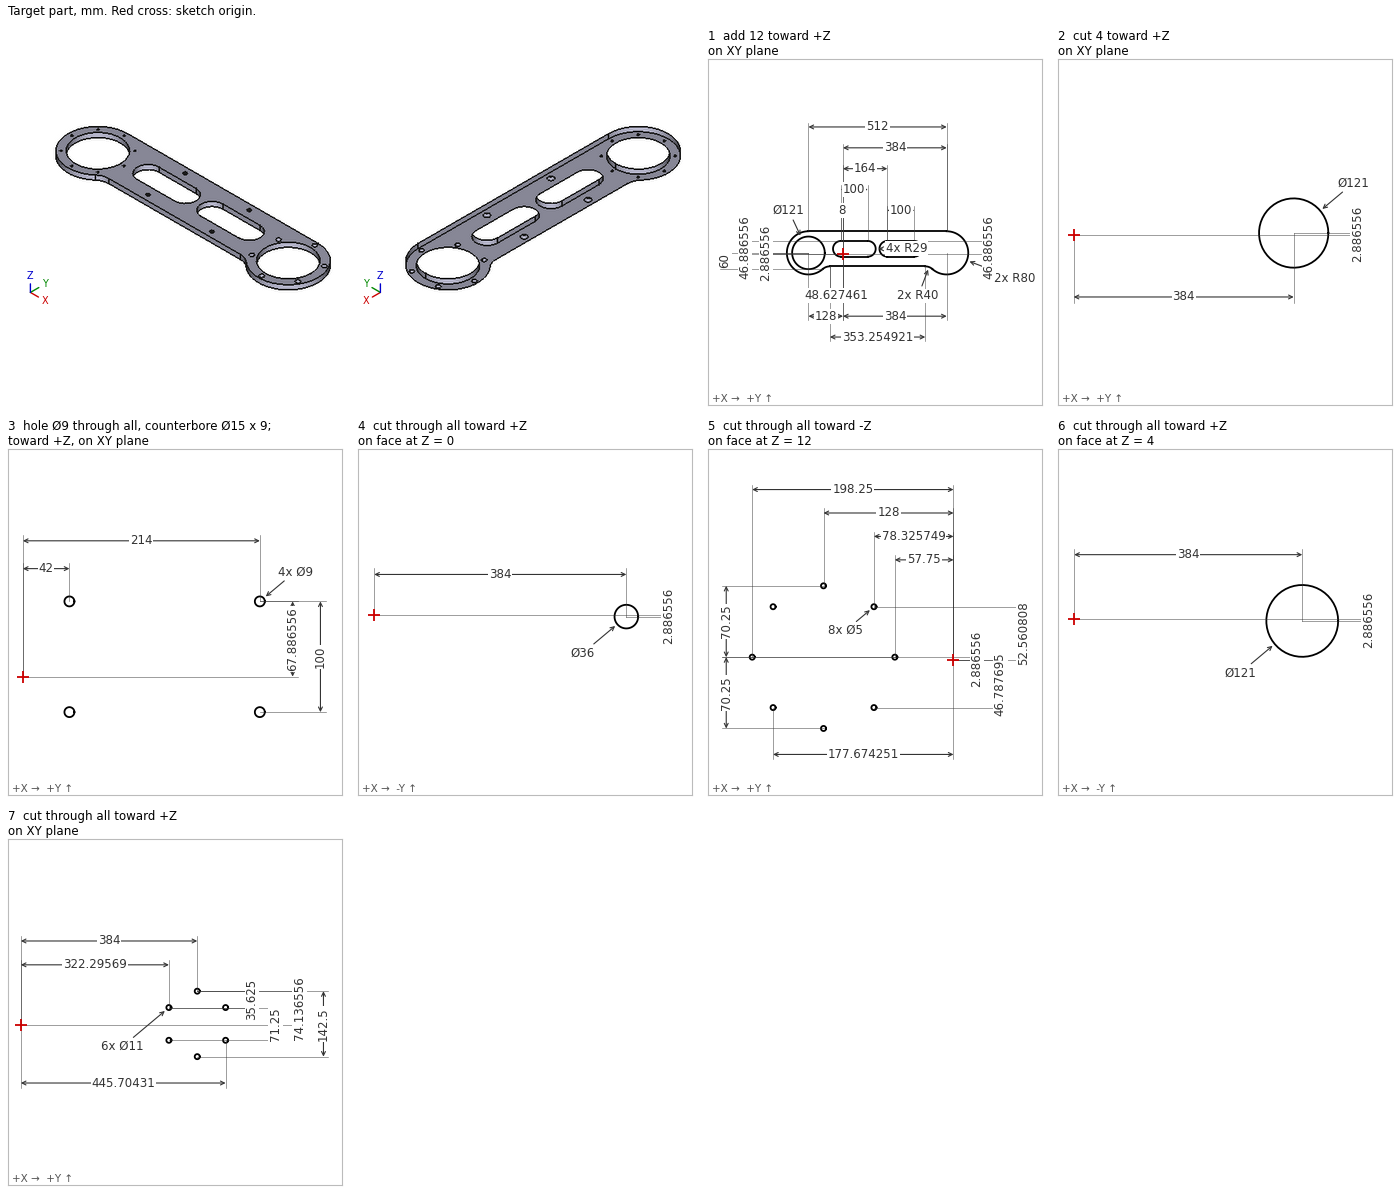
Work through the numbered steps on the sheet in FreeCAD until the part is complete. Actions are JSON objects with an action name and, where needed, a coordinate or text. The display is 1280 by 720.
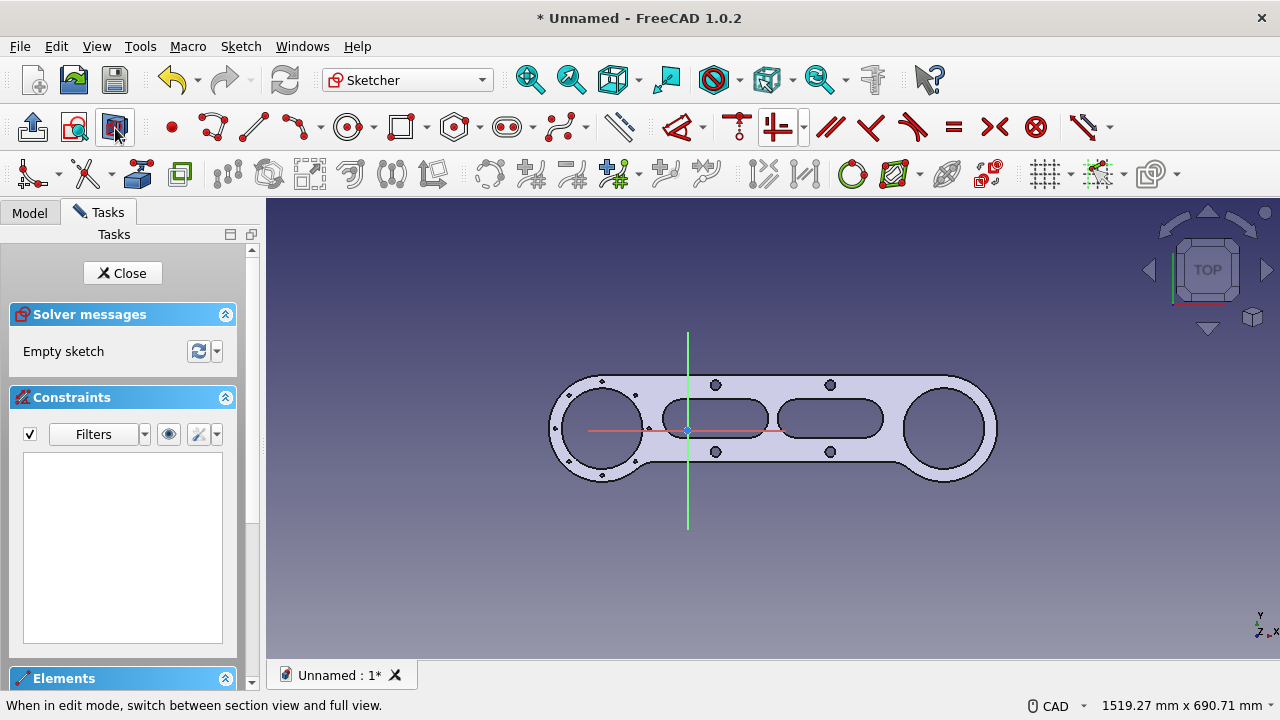
{"action": "scroll", "coordinate": [1083, 429], "scroll_direction": "up", "scroll_amount": 5}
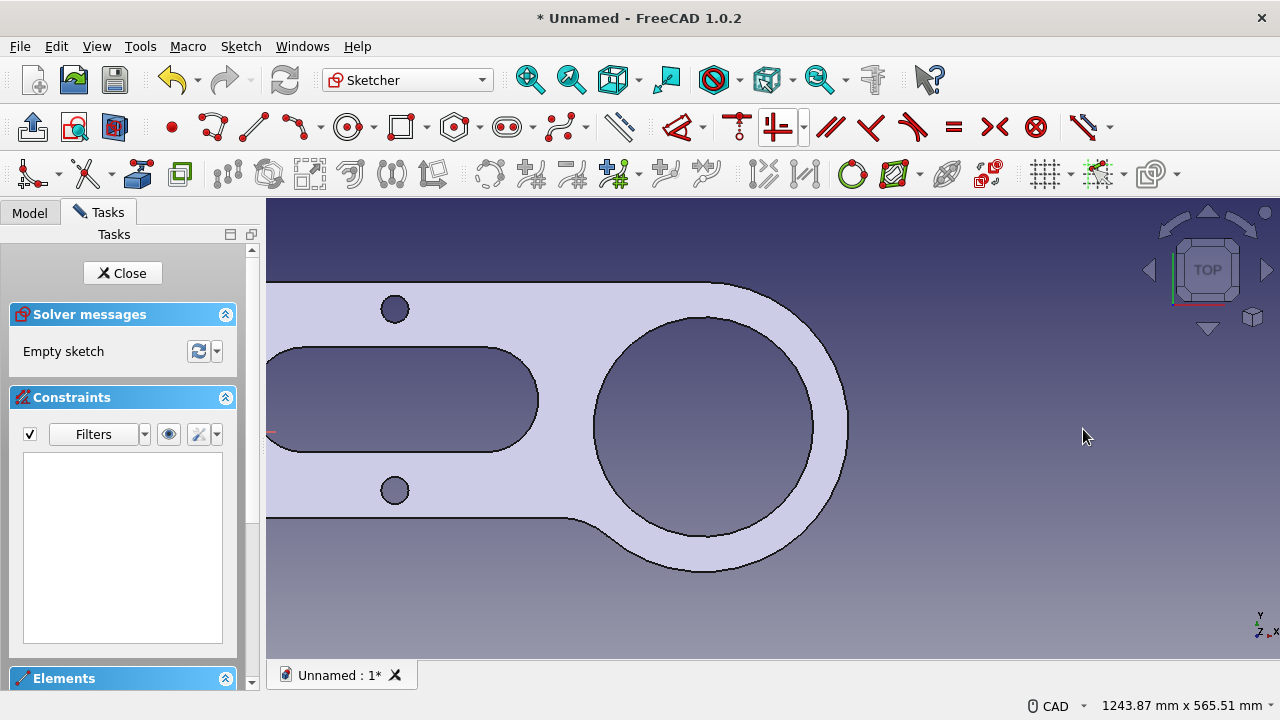
{"action": "left_click", "coordinate": [348, 128]}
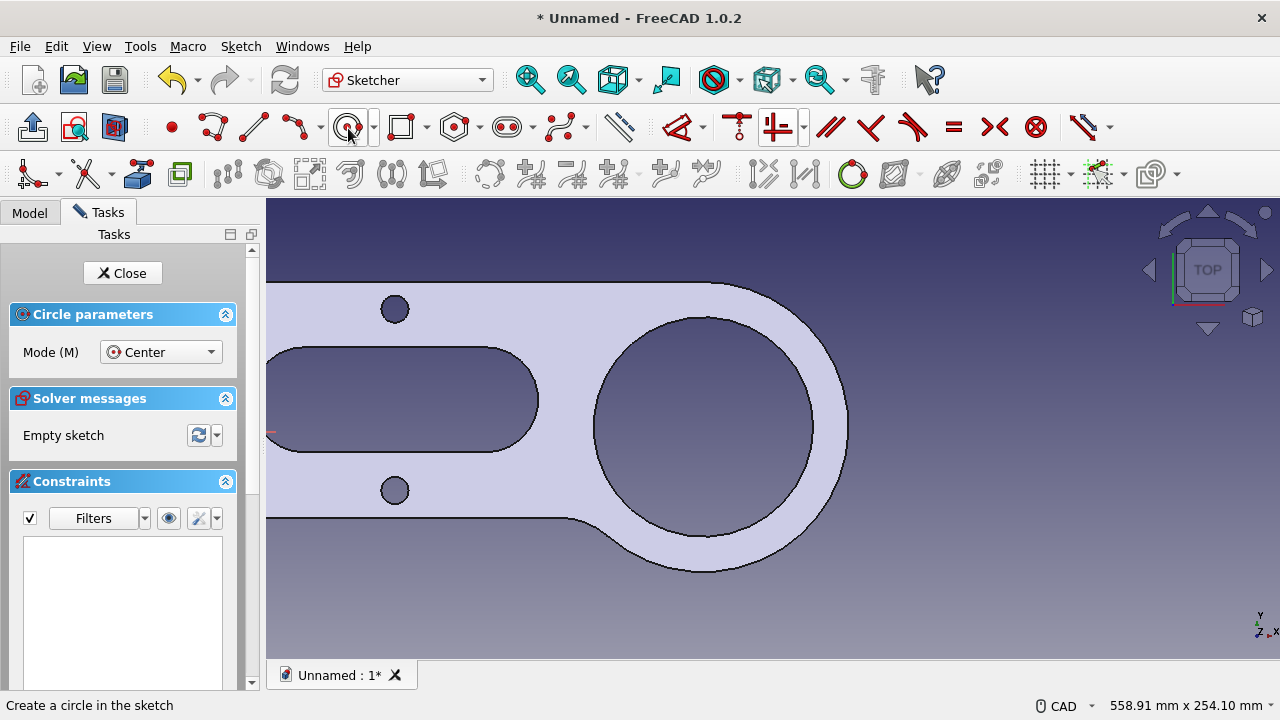
{"action": "scroll", "coordinate": [703, 298], "scroll_direction": "up", "scroll_amount": 5}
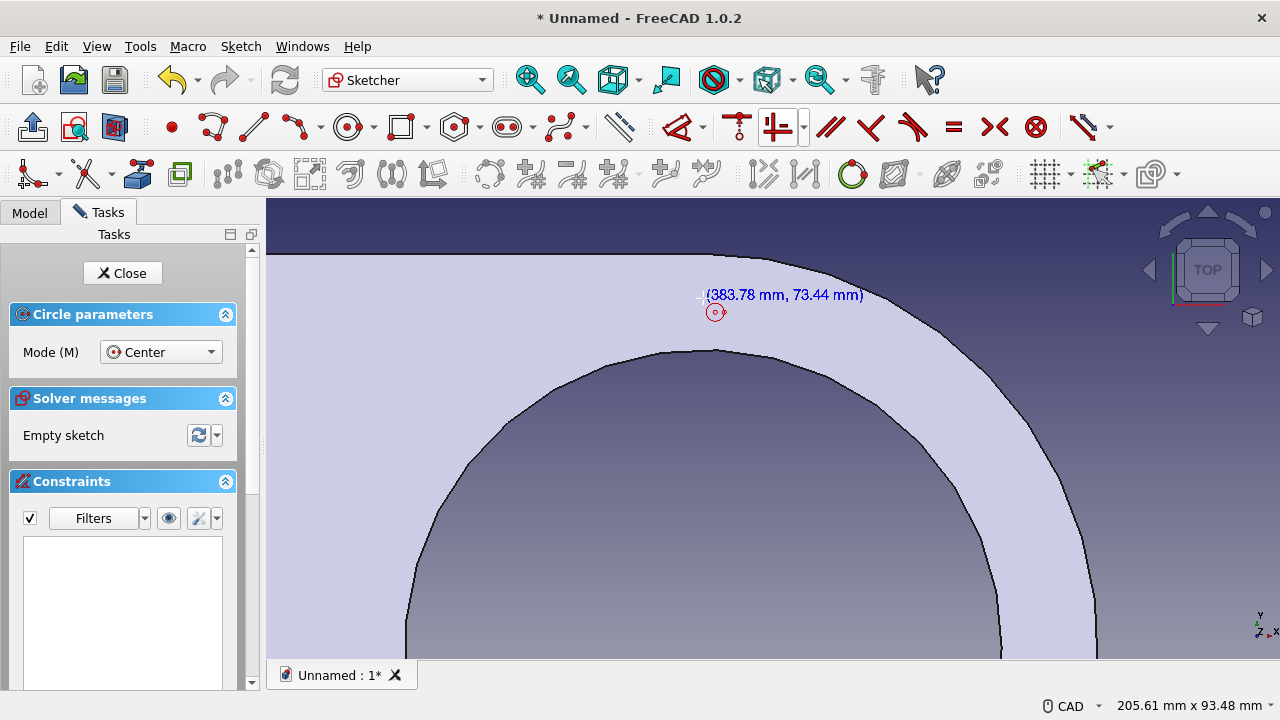
{"action": "left_click", "coordinate": [703, 297]}
{"action": "left_click", "coordinate": [723, 278]}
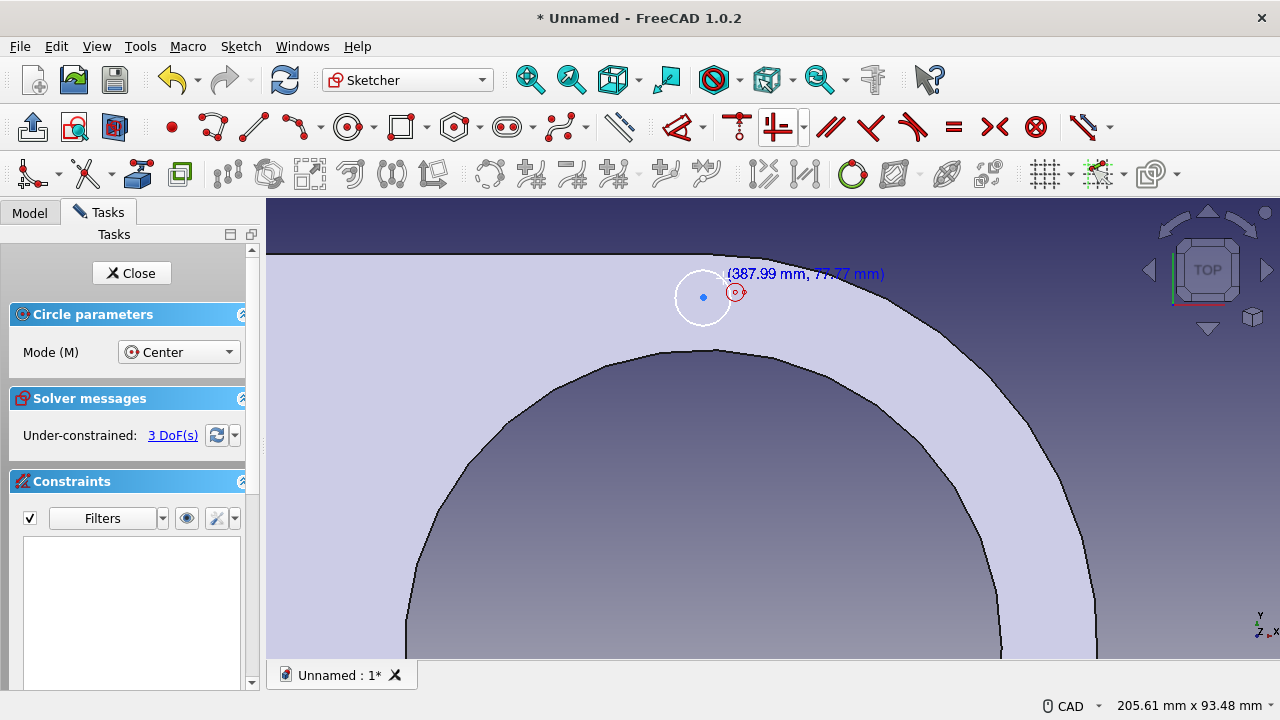
{"action": "left_click", "coordinate": [399, 473]}
{"action": "left_click", "coordinate": [418, 453]}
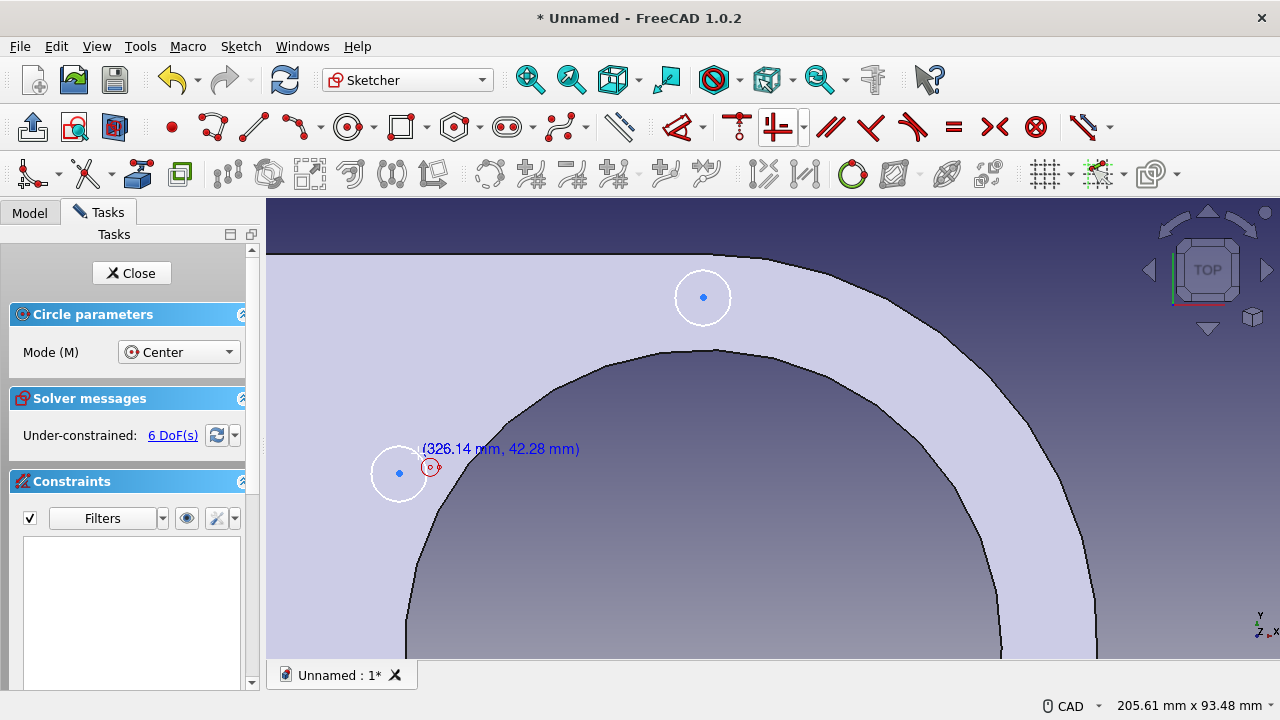
{"action": "scroll", "coordinate": [705, 301], "scroll_direction": "down", "scroll_amount": 5}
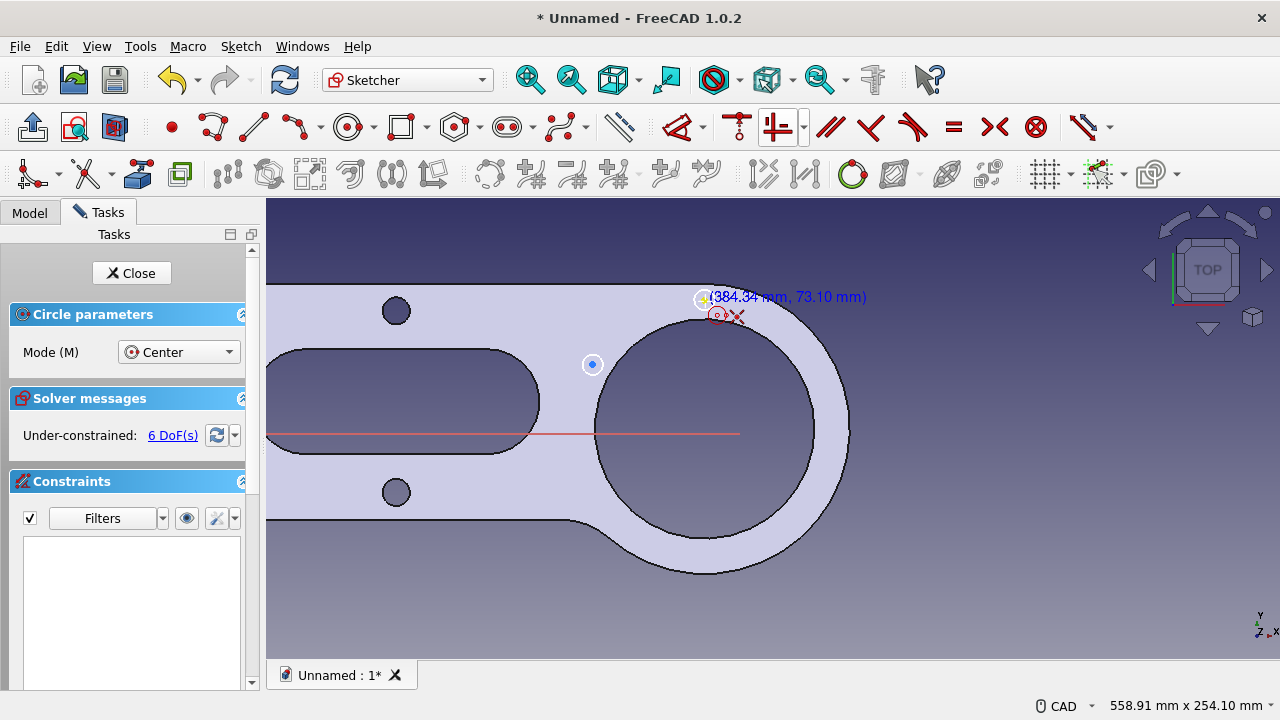
{"action": "scroll", "coordinate": [593, 494], "scroll_direction": "up", "scroll_amount": 5}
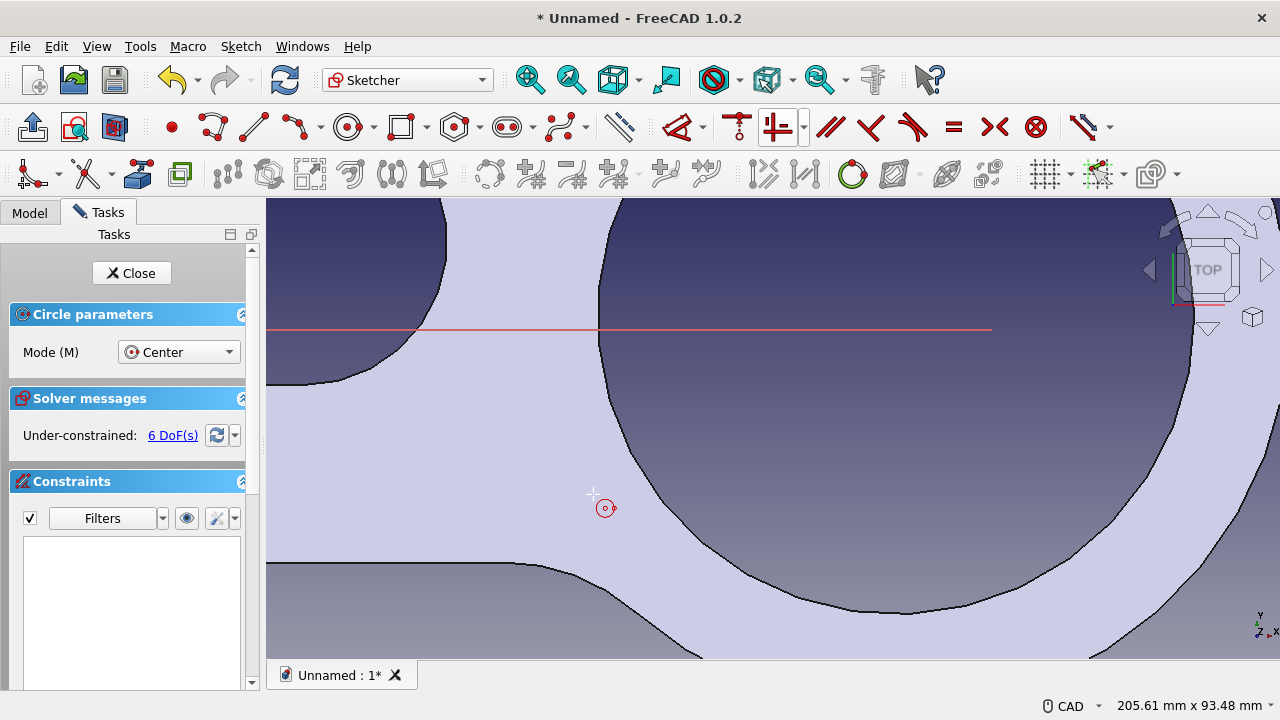
{"action": "left_click", "coordinate": [592, 492]}
{"action": "left_click", "coordinate": [611, 472]}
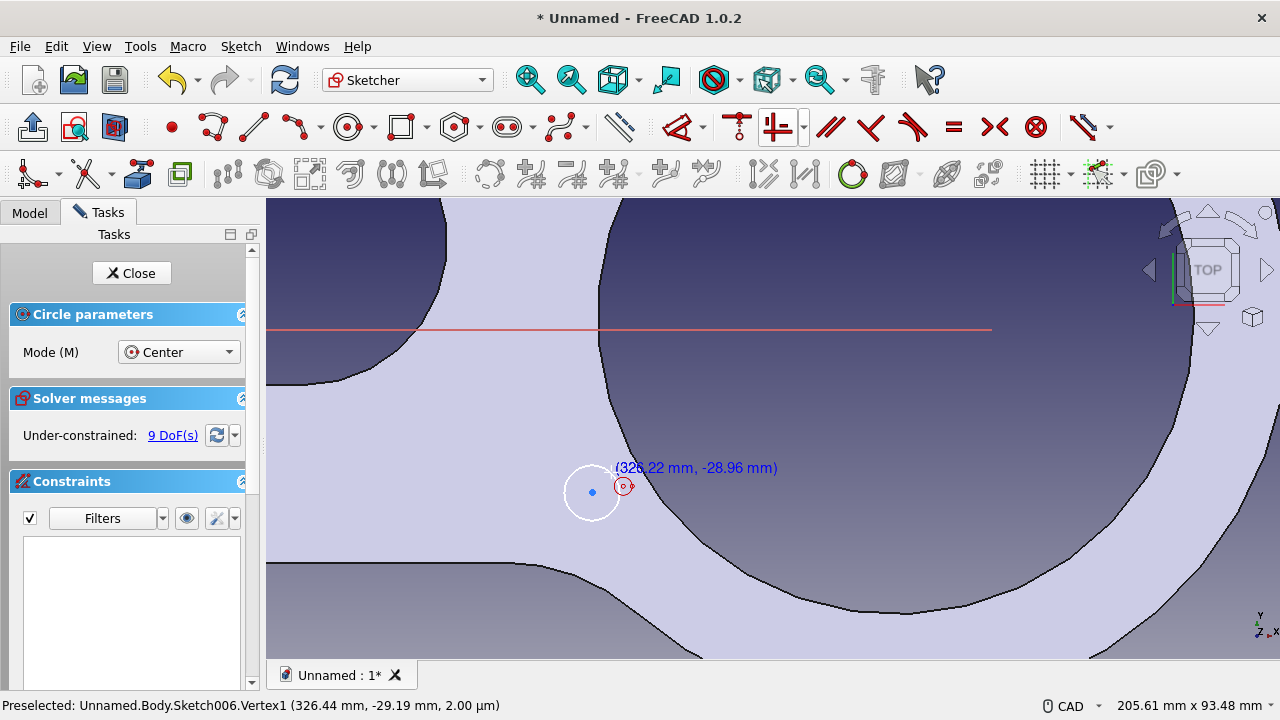
{"action": "scroll", "coordinate": [593, 494], "scroll_direction": "down", "scroll_amount": 5}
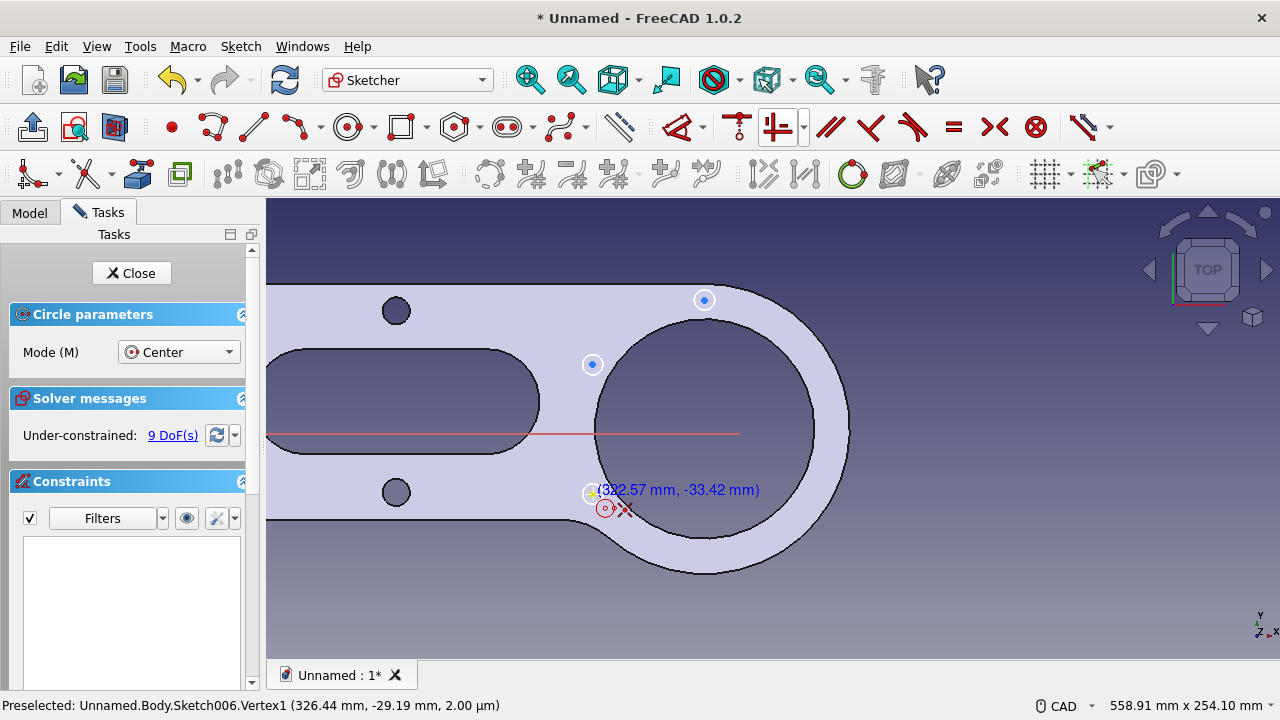
{"action": "scroll", "coordinate": [705, 558], "scroll_direction": "up", "scroll_amount": 5}